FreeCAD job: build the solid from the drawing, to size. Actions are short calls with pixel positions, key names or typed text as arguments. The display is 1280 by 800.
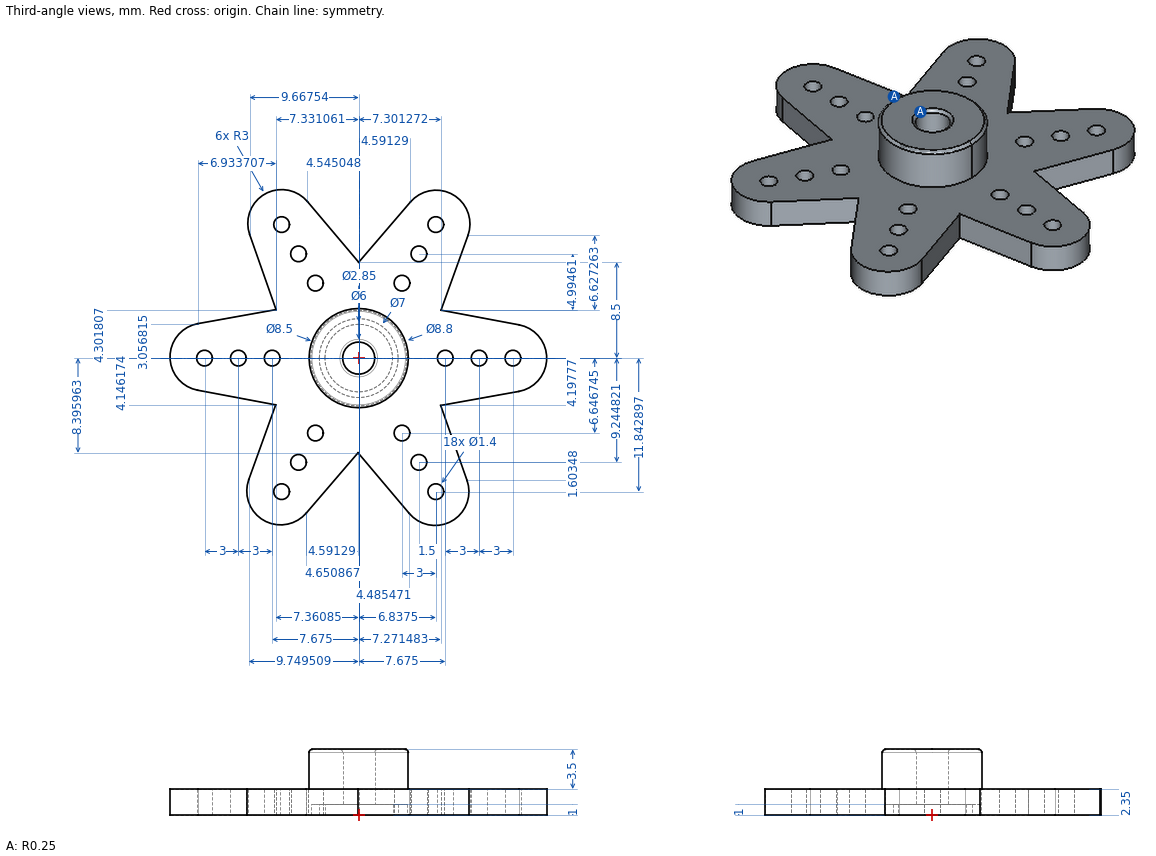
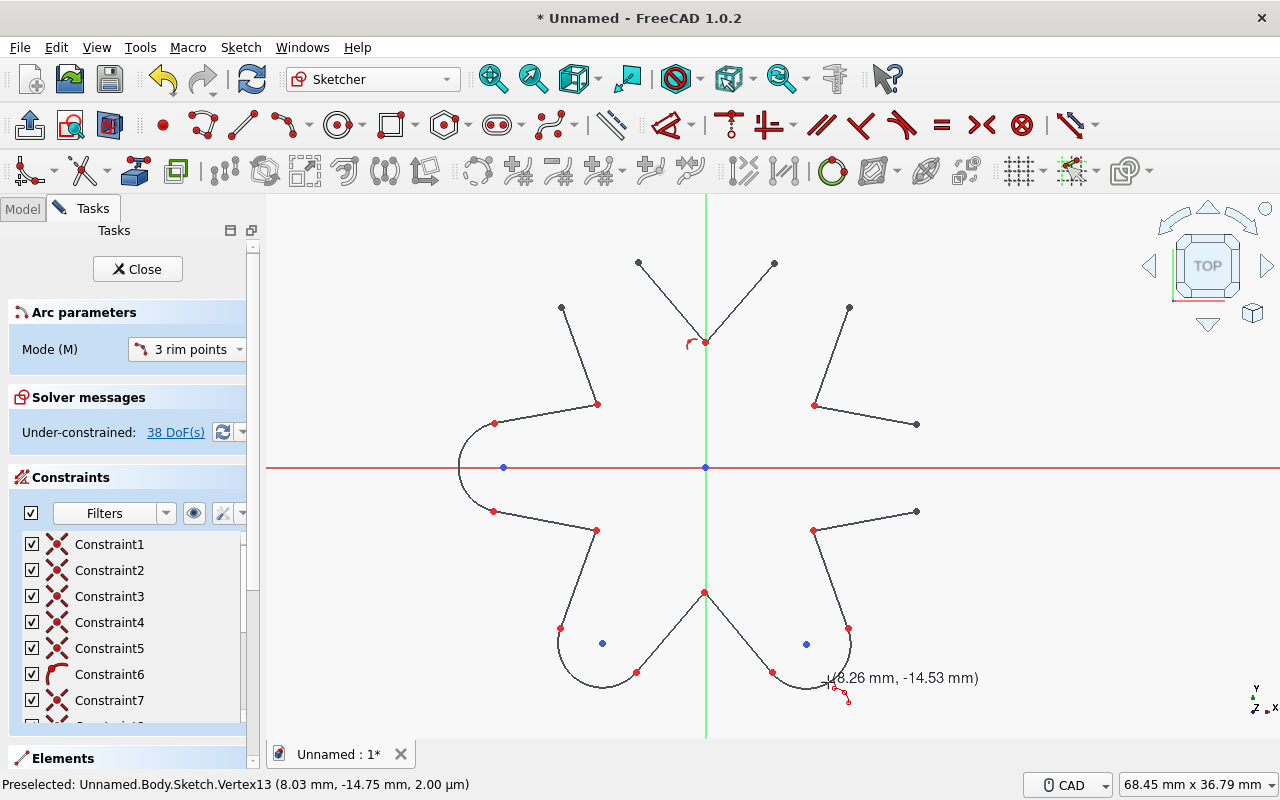
click(916, 512)
click(916, 425)
click(946, 491)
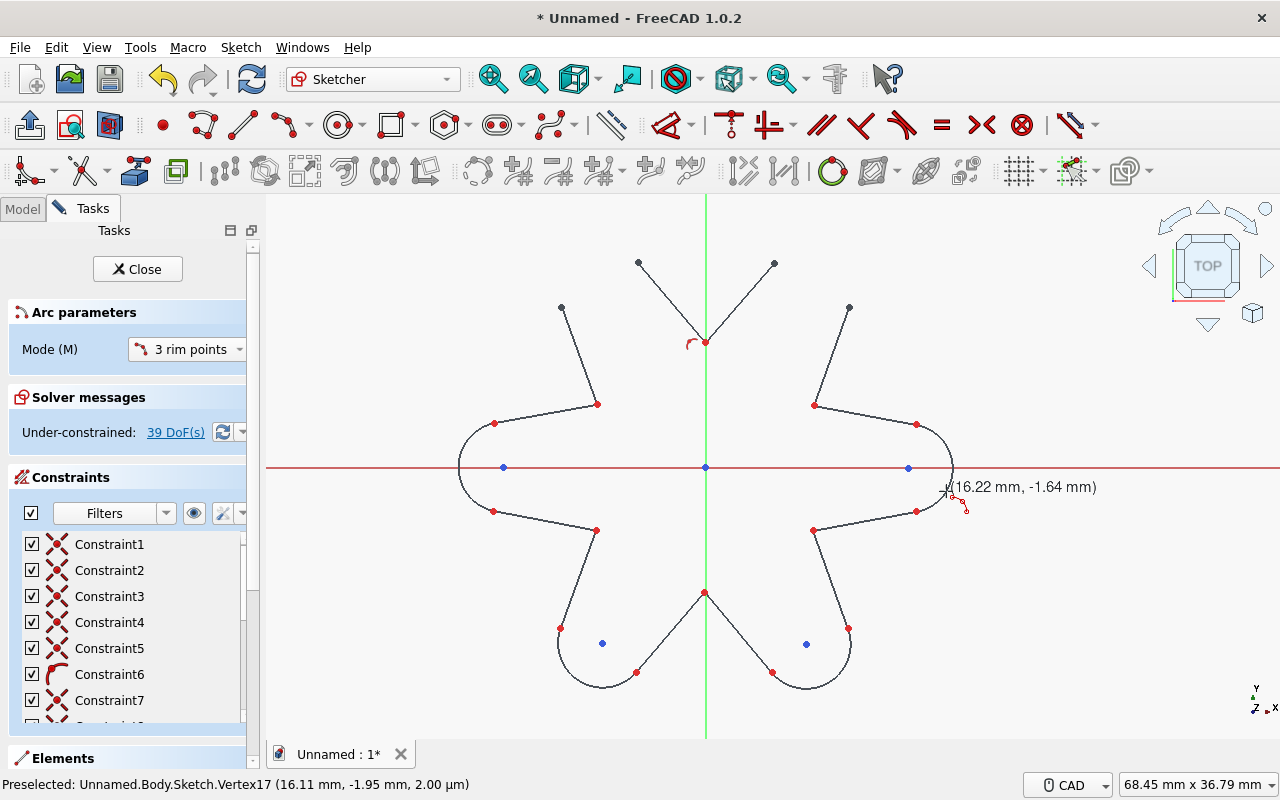
click(849, 308)
click(774, 264)
click(830, 253)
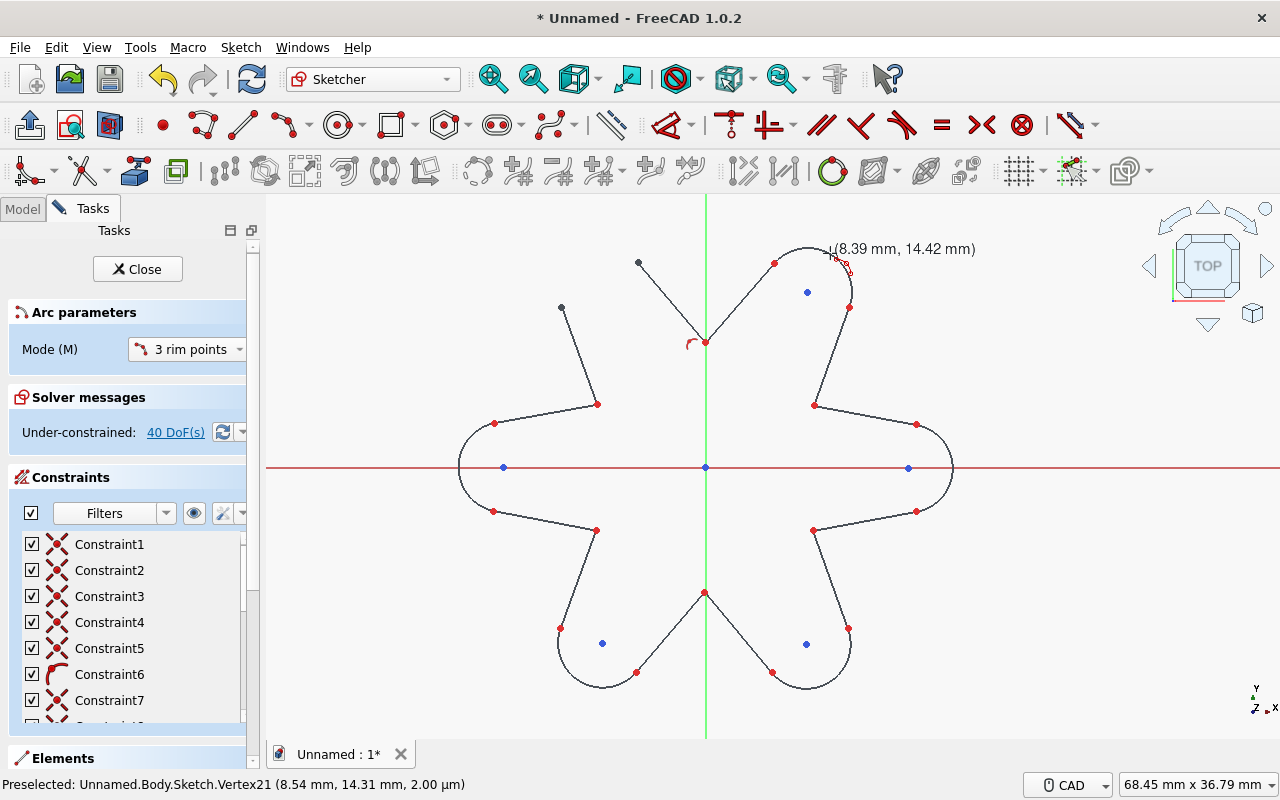
click(638, 263)
click(562, 307)
click(582, 252)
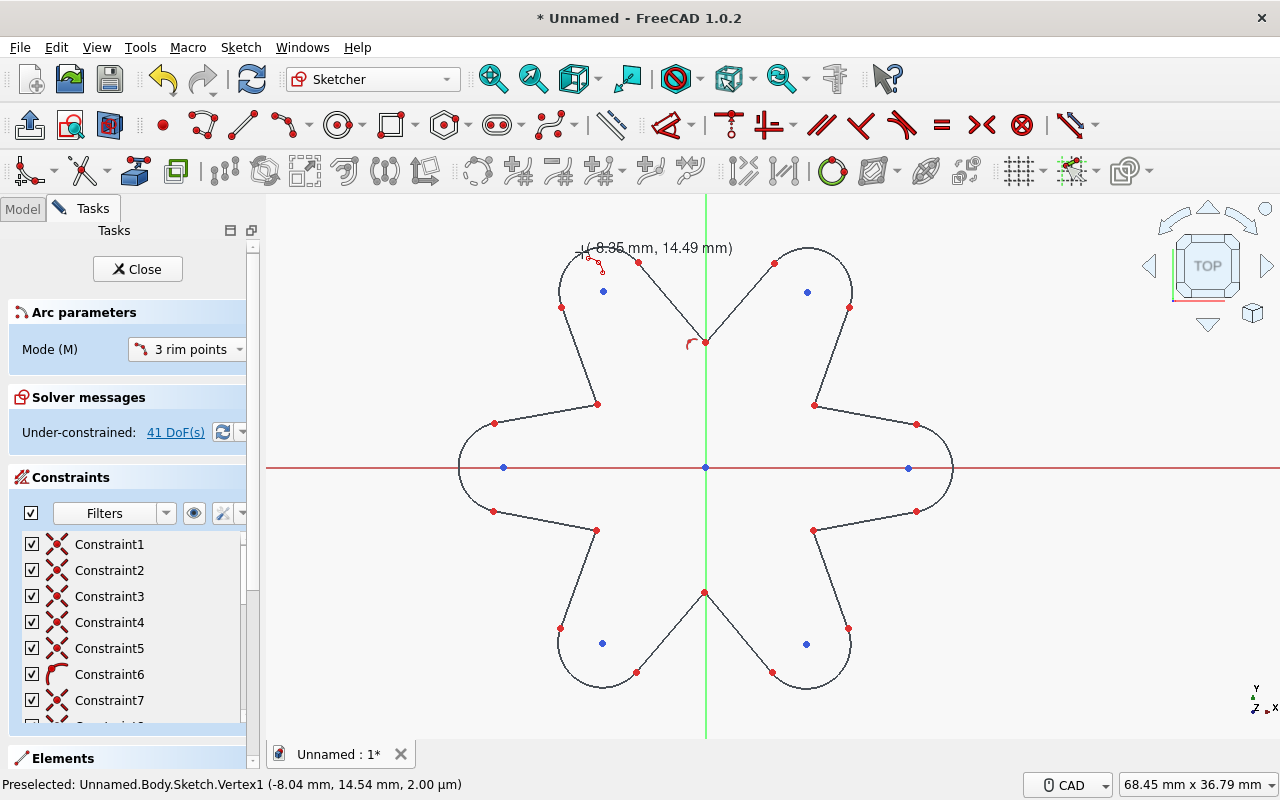
click(338, 126)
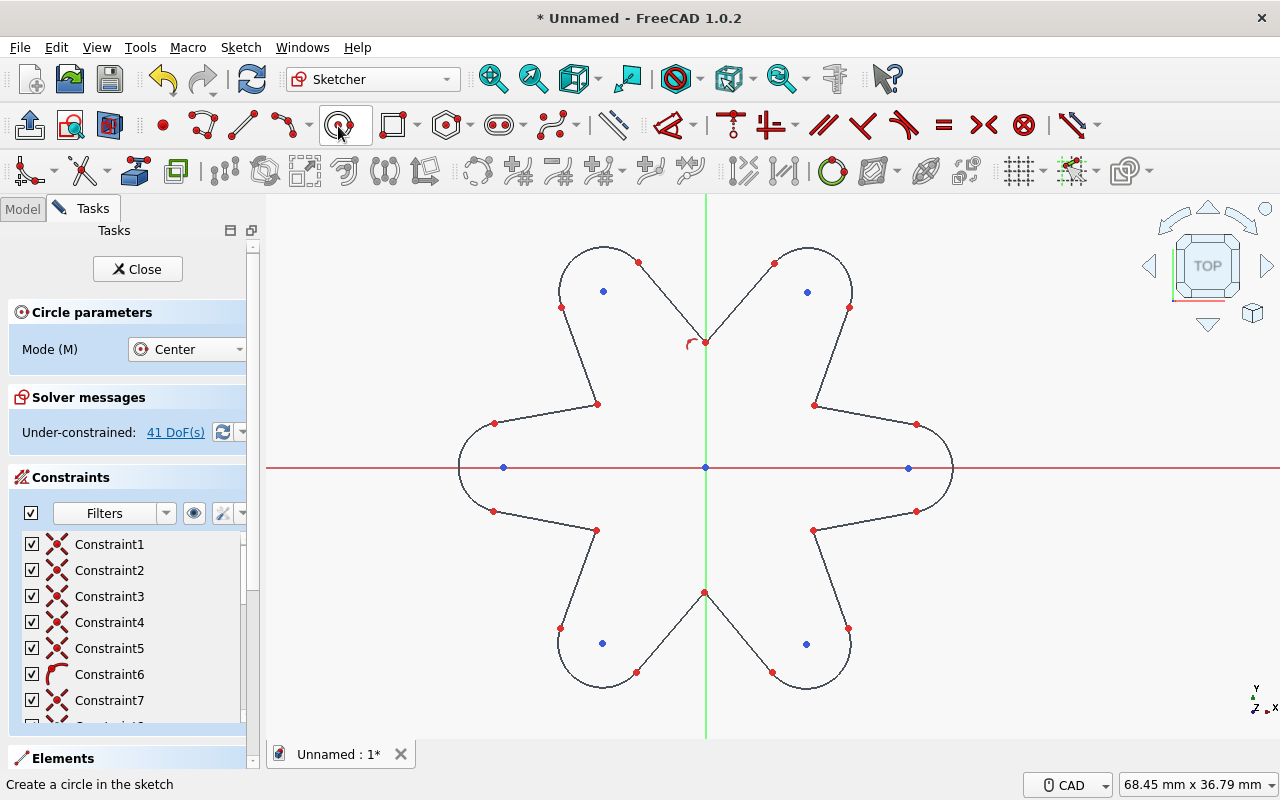
scroll(807, 643, up, 15)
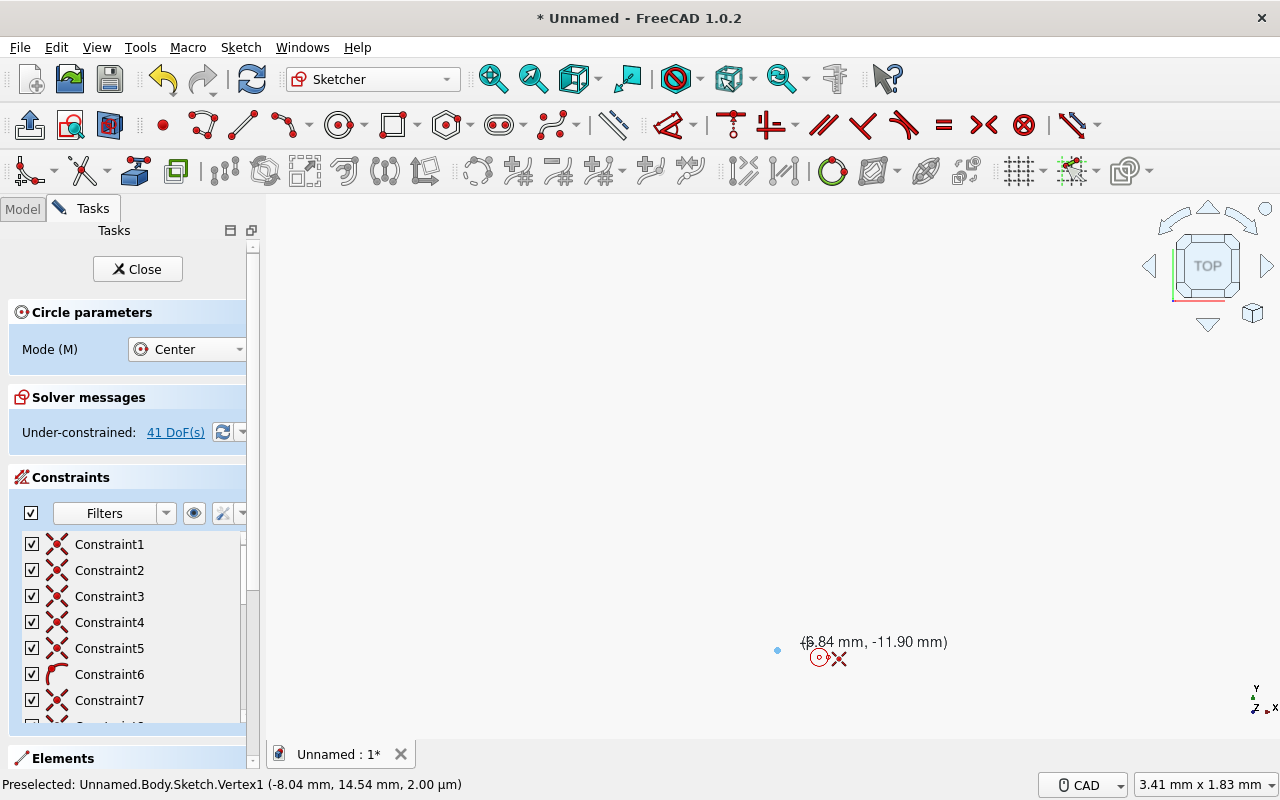
click(796, 630)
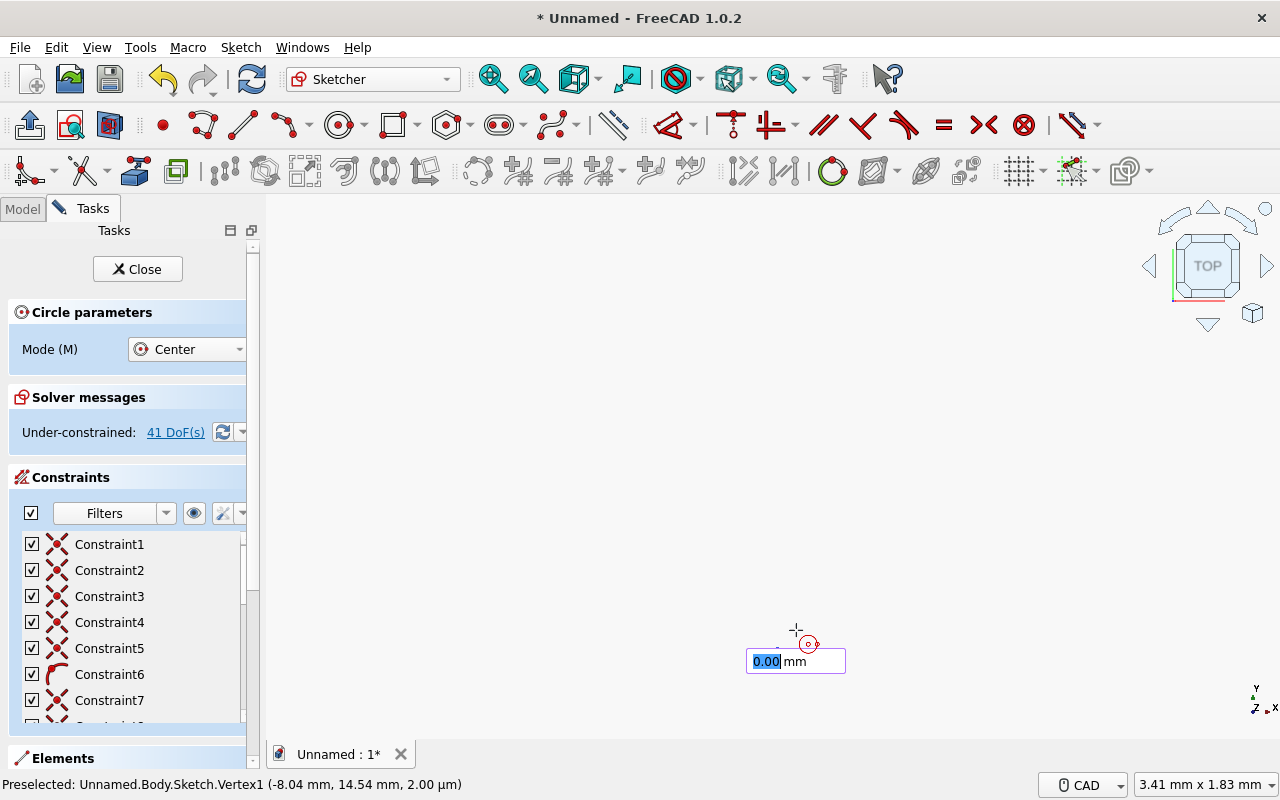
scroll(807, 643, down, 15)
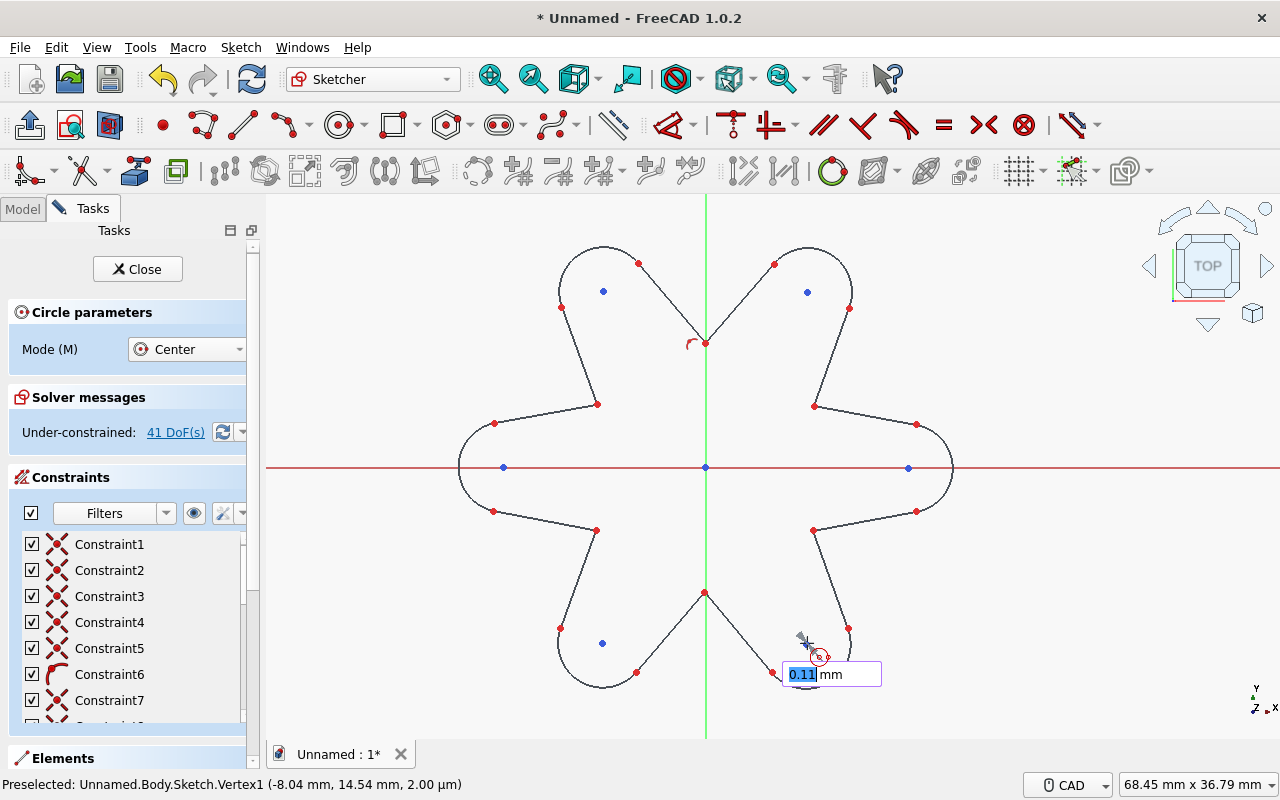
scroll(814, 636, up, 3)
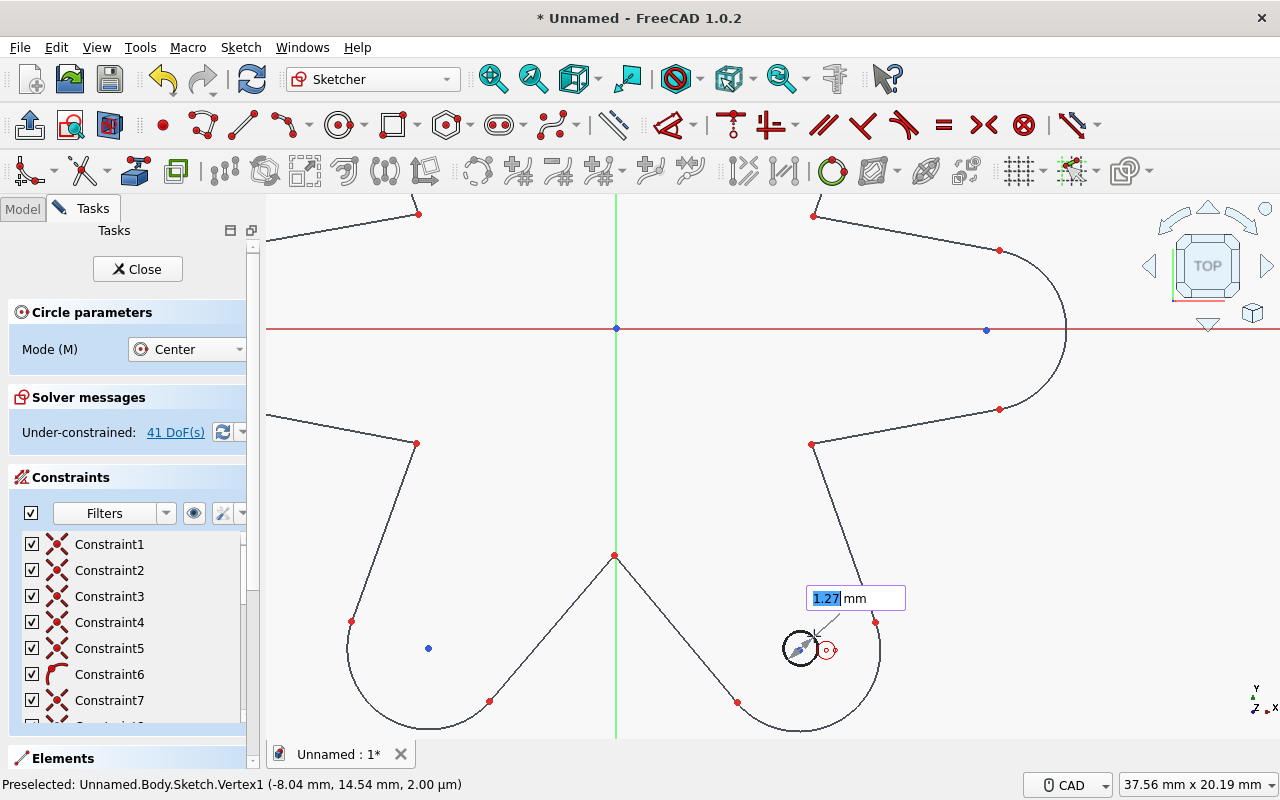
click(814, 635)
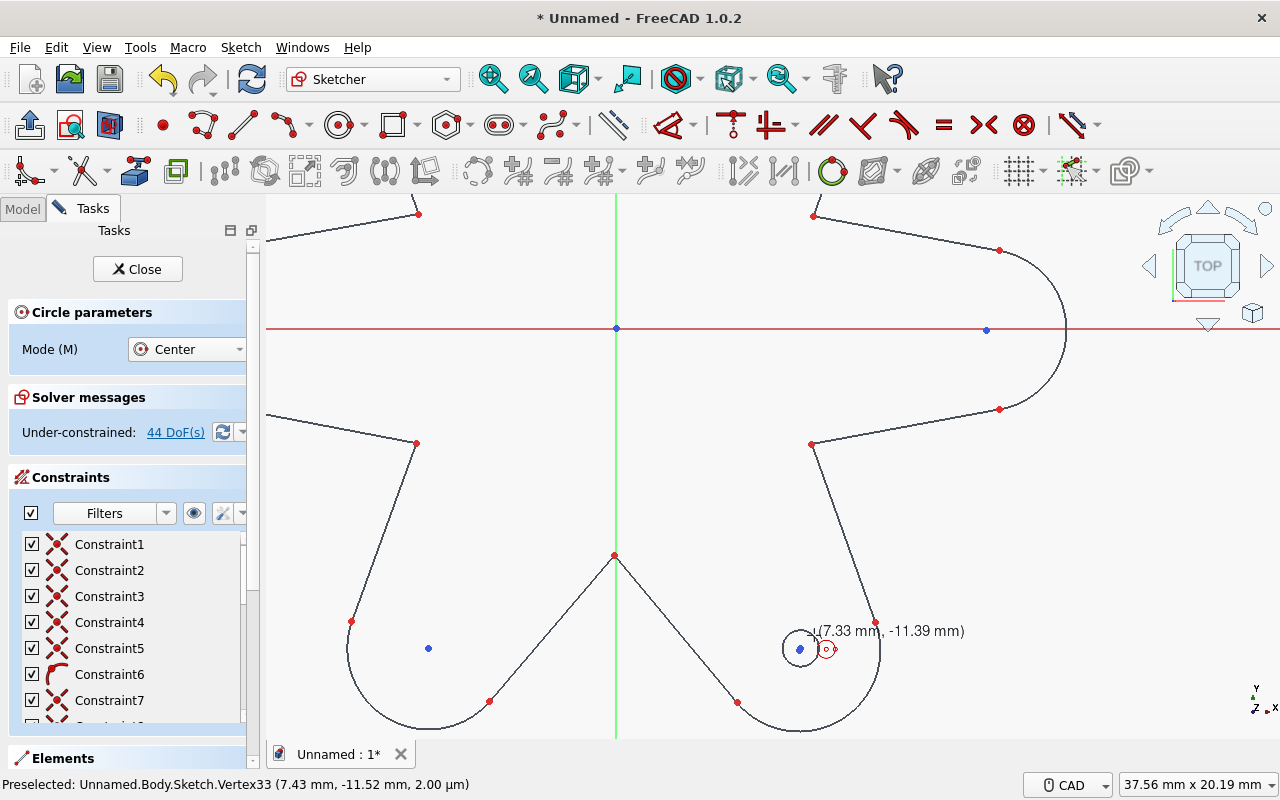
click(760, 578)
click(774, 565)